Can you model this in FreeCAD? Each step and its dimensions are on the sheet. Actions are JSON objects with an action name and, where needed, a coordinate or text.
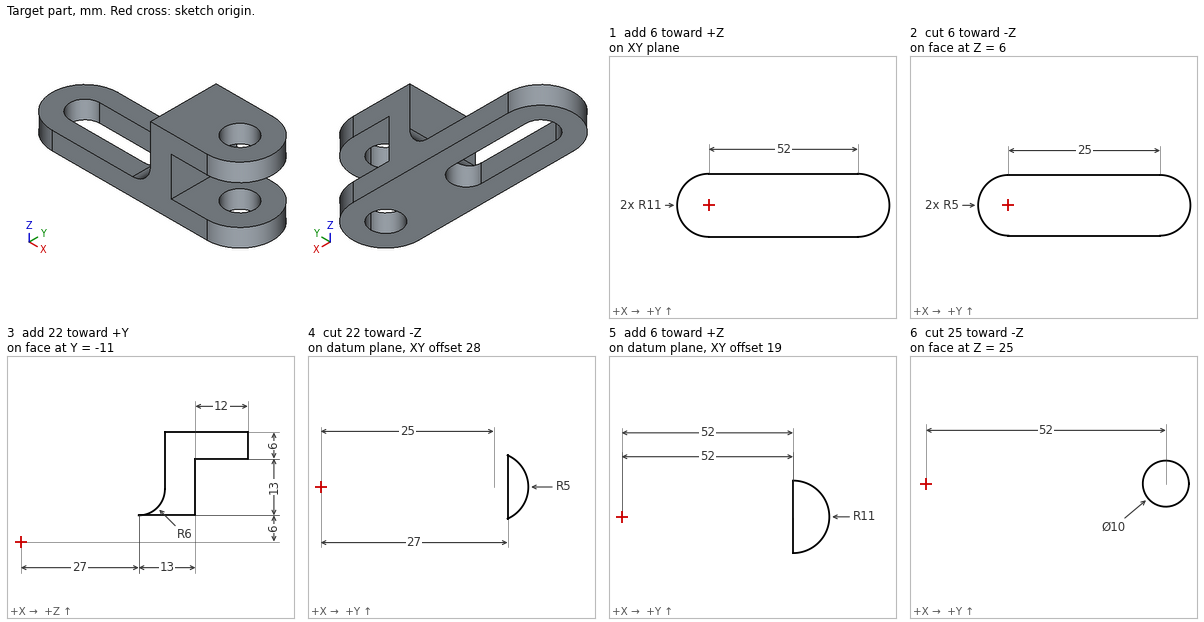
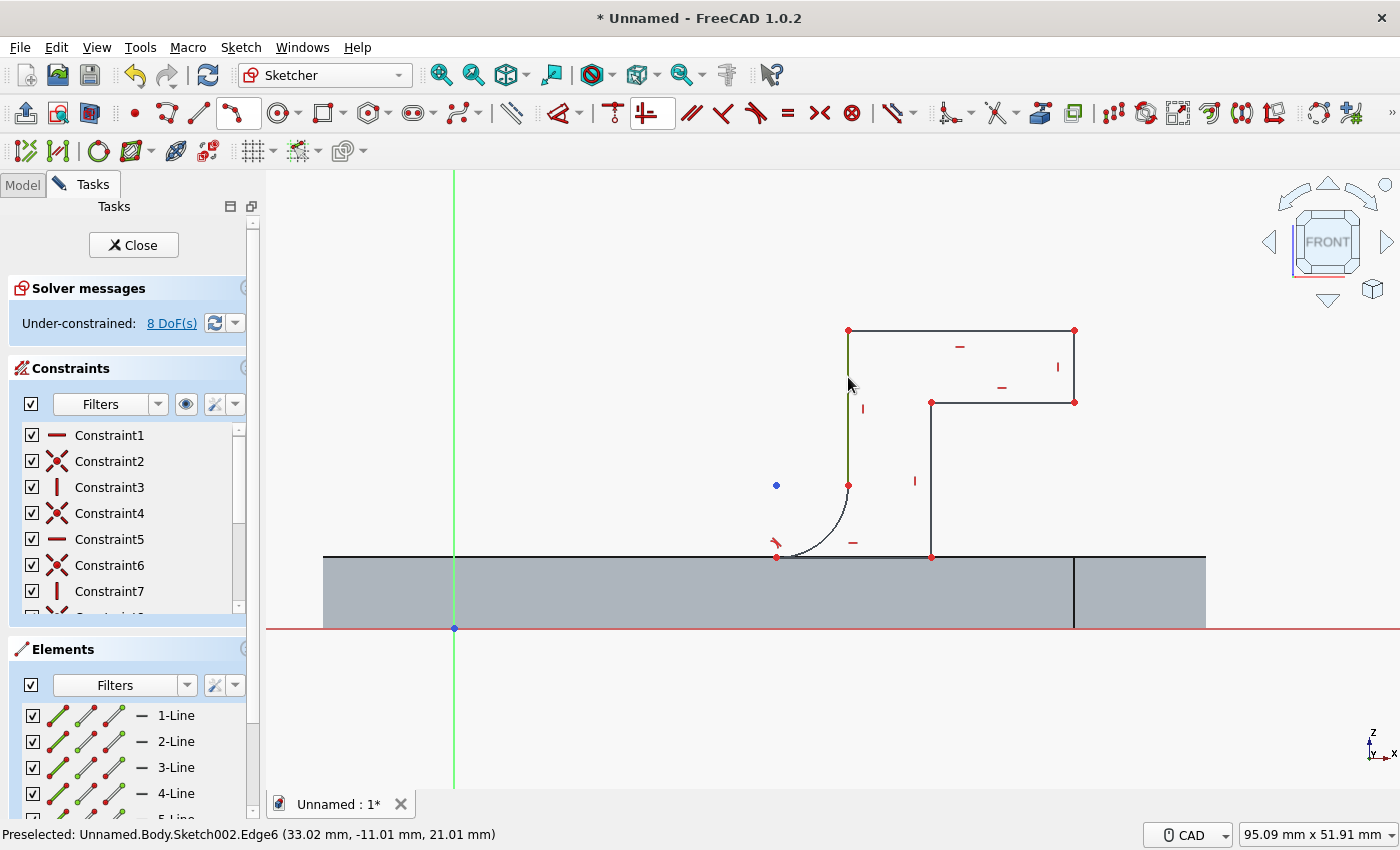
{"action": "left_click", "coordinate": [840, 519]}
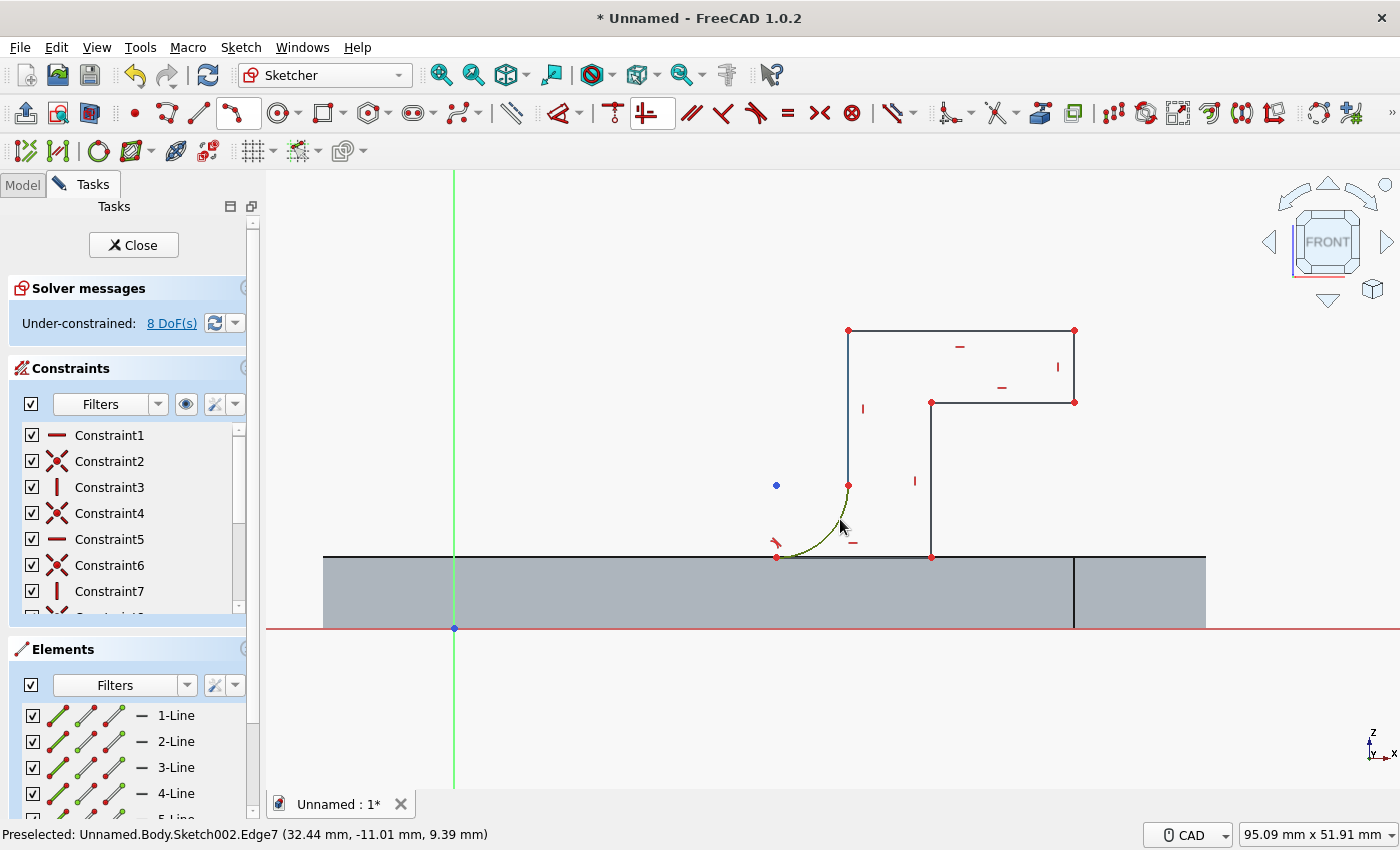
{"action": "left_click", "coordinate": [756, 114]}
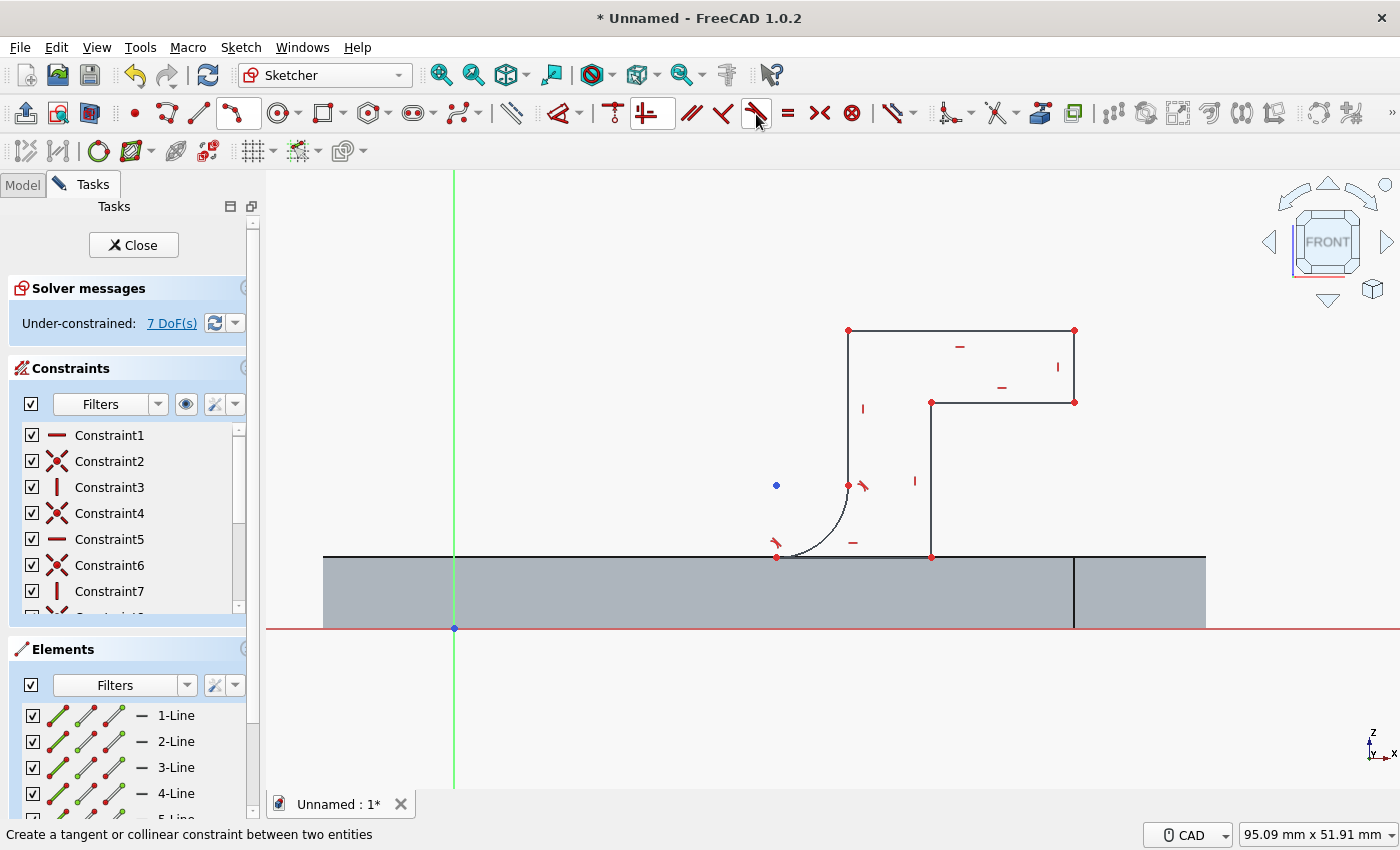
{"action": "key", "text": "d"}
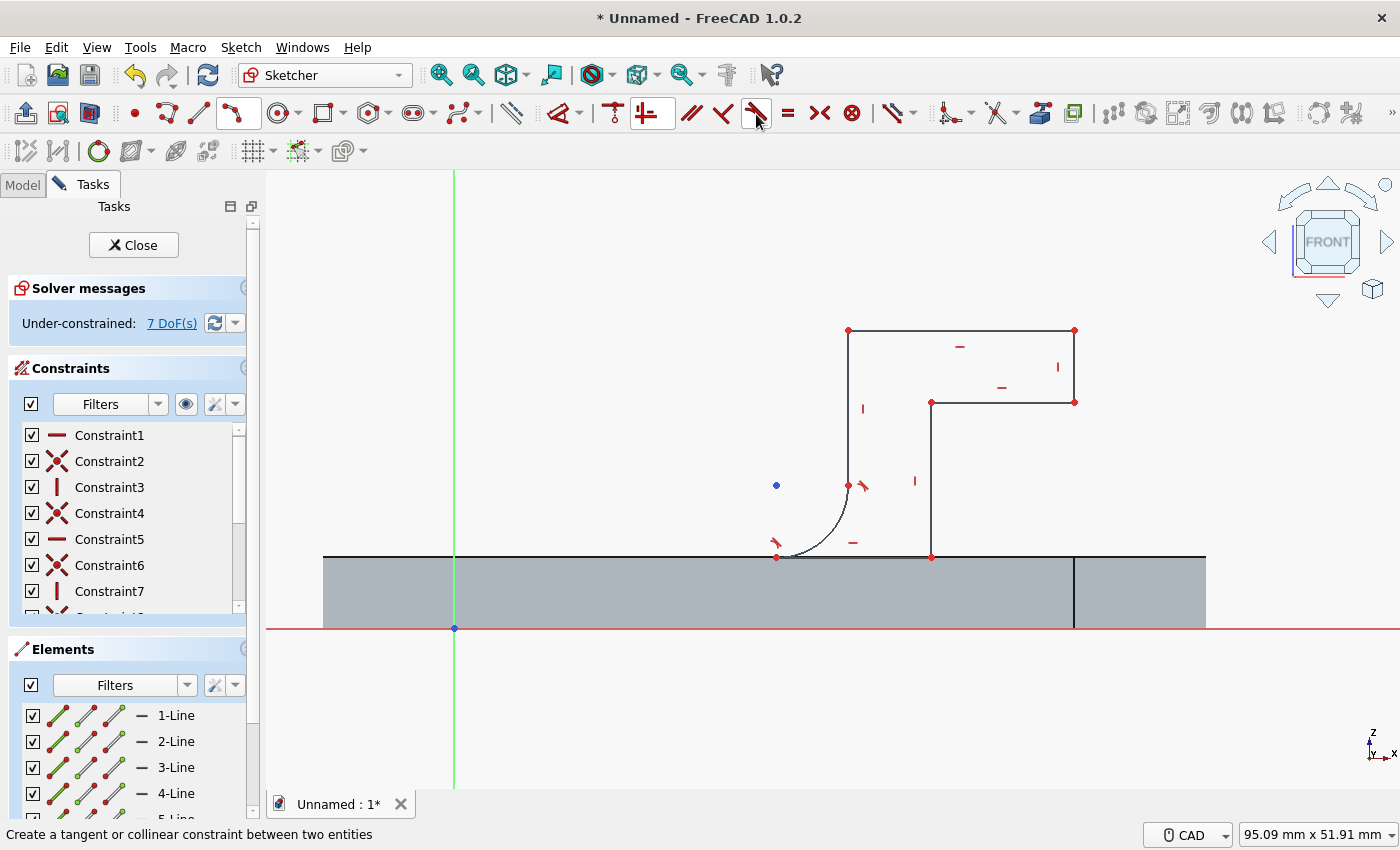
{"action": "left_click", "coordinate": [840, 519]}
{"action": "left_click", "coordinate": [868, 534]}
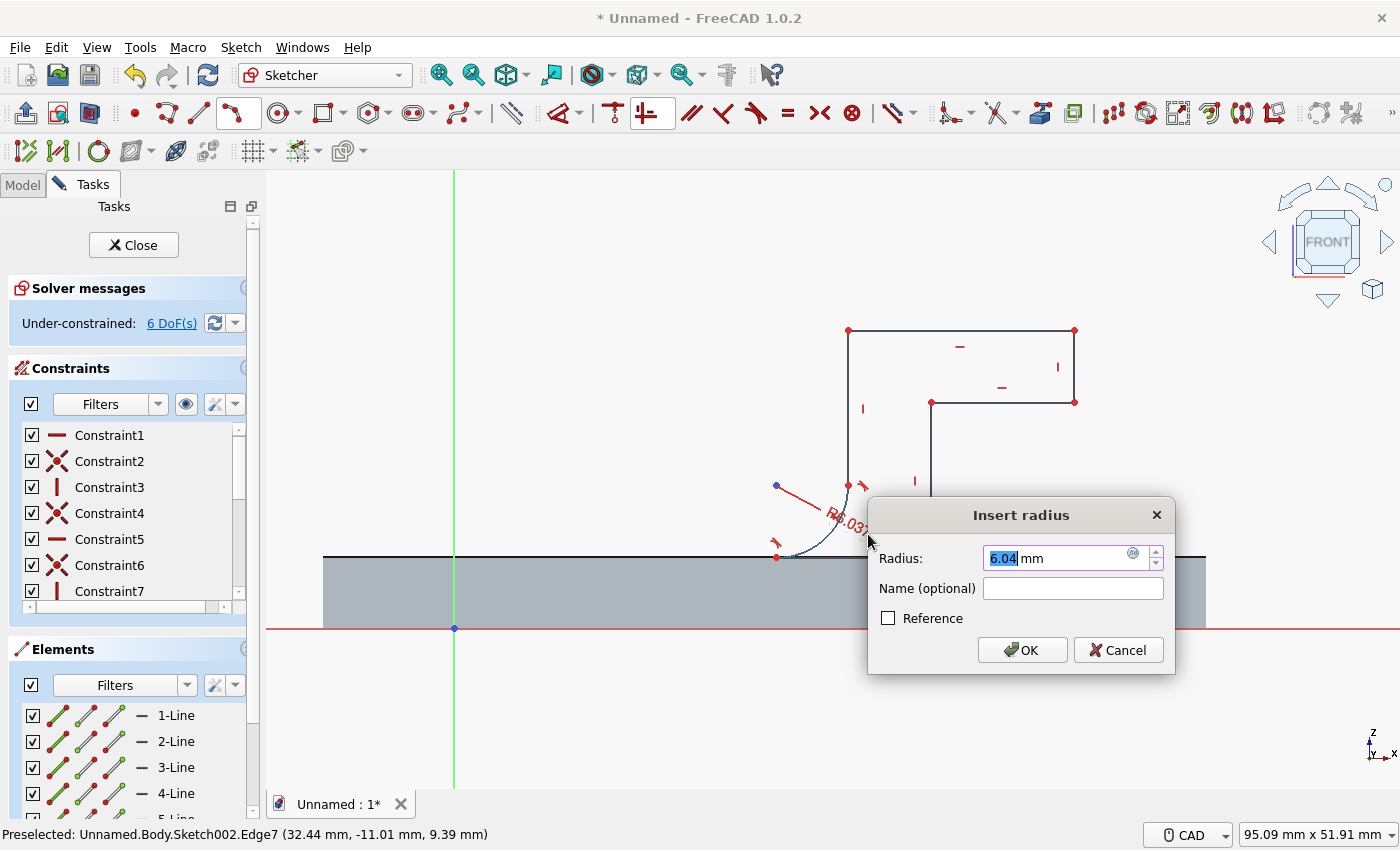
{"action": "type", "text": "6"}
{"action": "key", "text": "Return"}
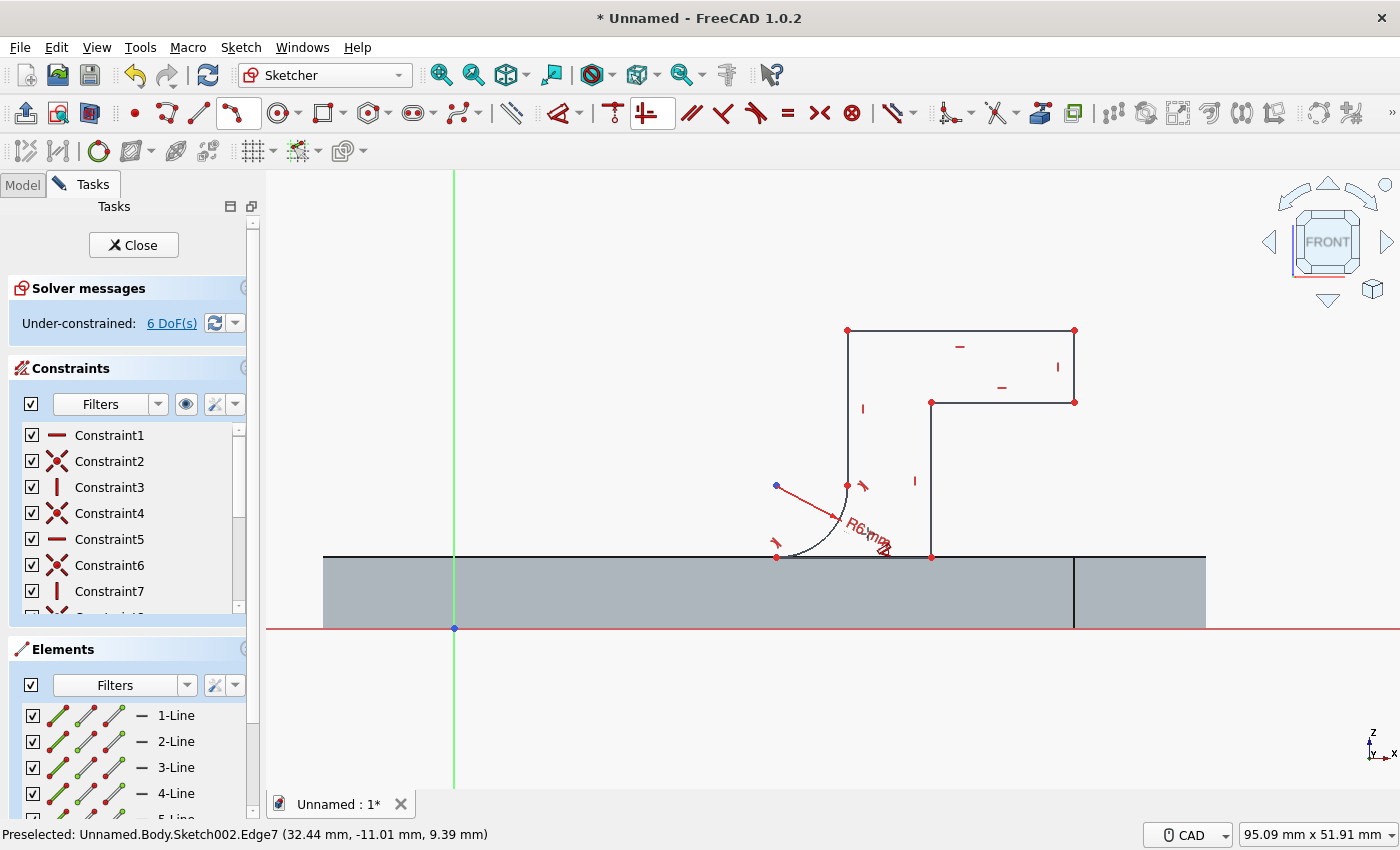
{"action": "left_click", "coordinate": [1074, 381]}
{"action": "left_click", "coordinate": [1108, 367]}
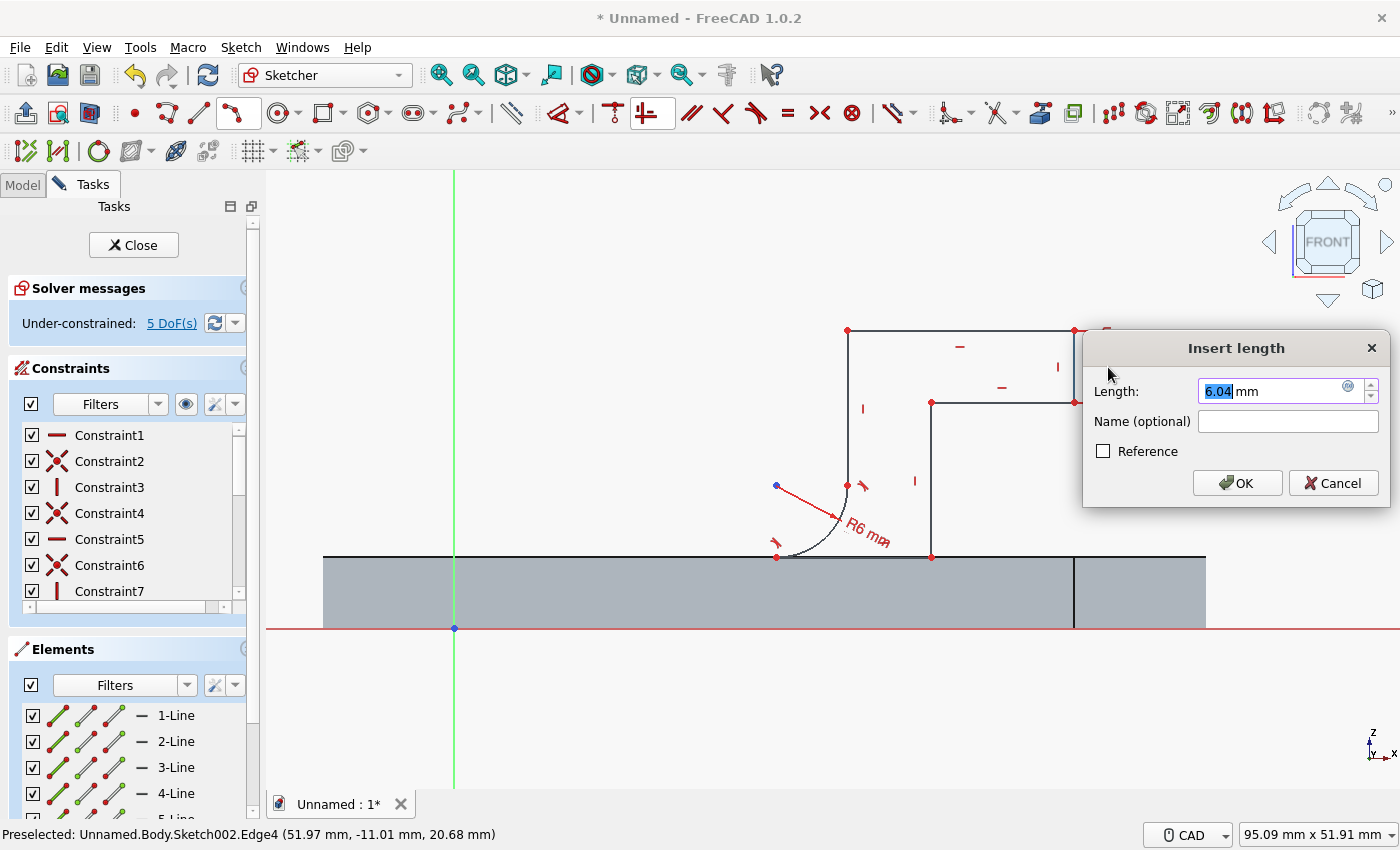
{"action": "type", "text": "6"}
{"action": "key", "text": "Return"}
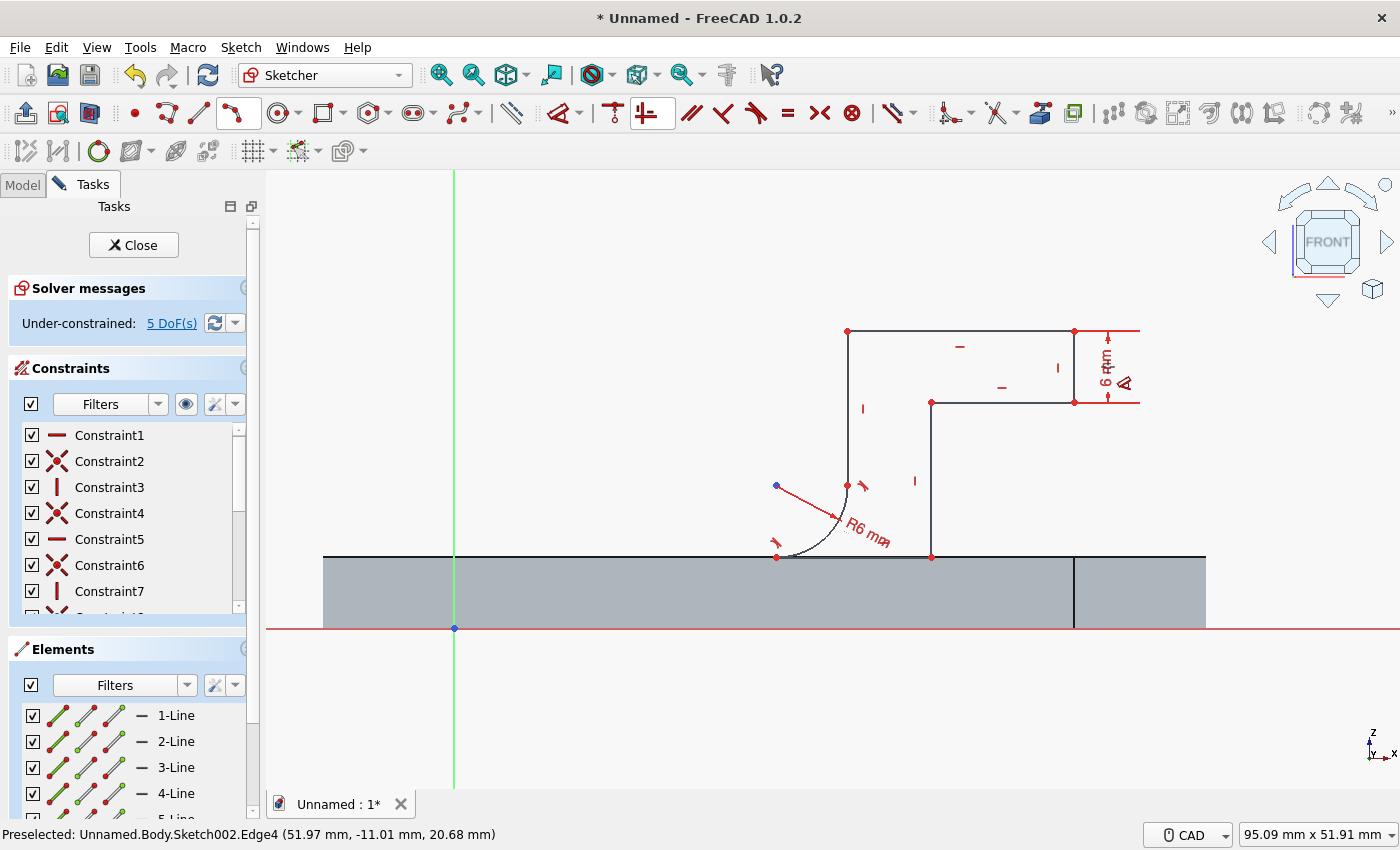
{"action": "left_click", "coordinate": [823, 558]}
{"action": "left_click", "coordinate": [854, 592]}